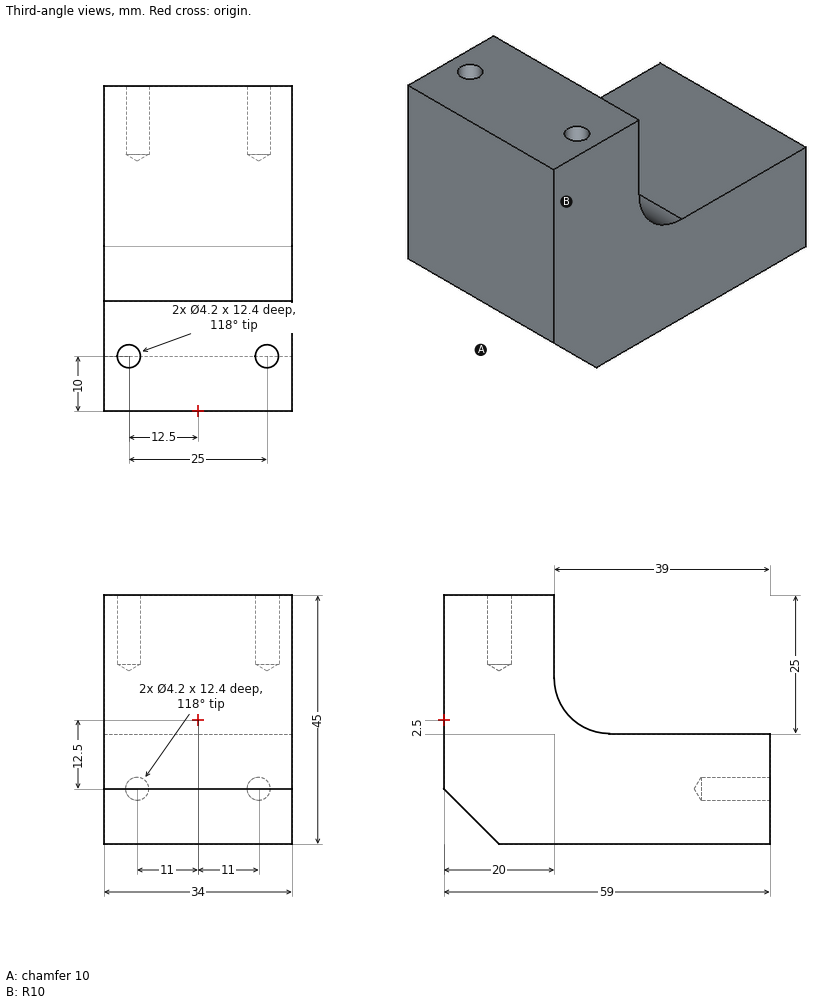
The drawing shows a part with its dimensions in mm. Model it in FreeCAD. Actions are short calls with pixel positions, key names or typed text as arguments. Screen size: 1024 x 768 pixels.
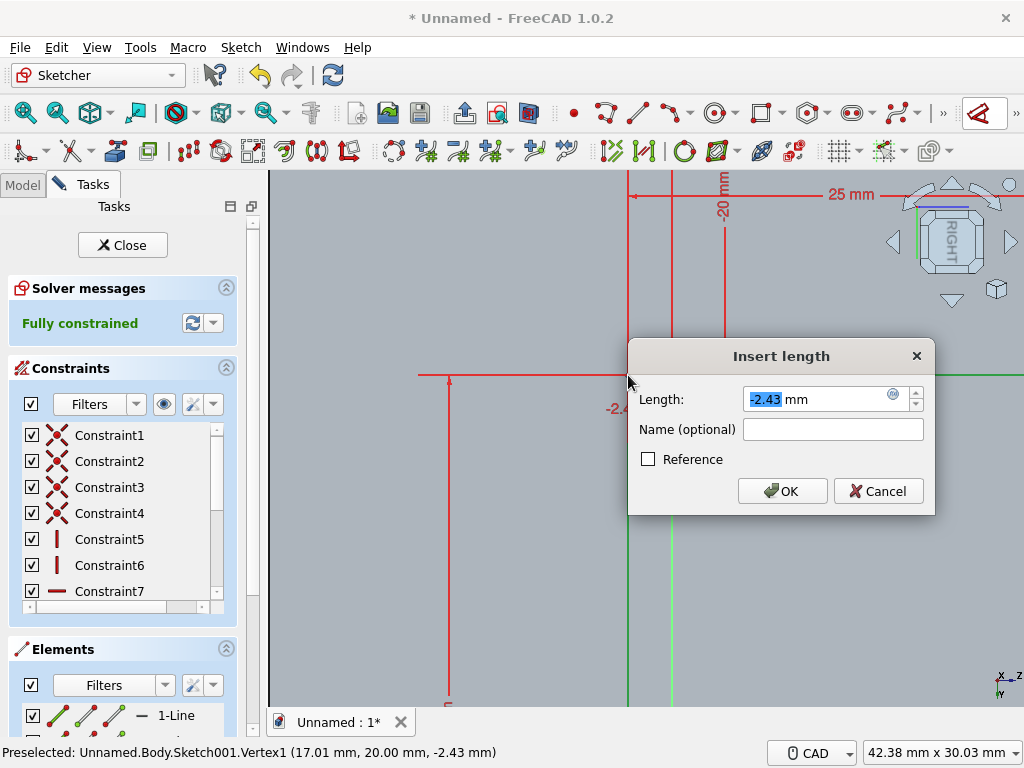
text(-2.5)
key(Return)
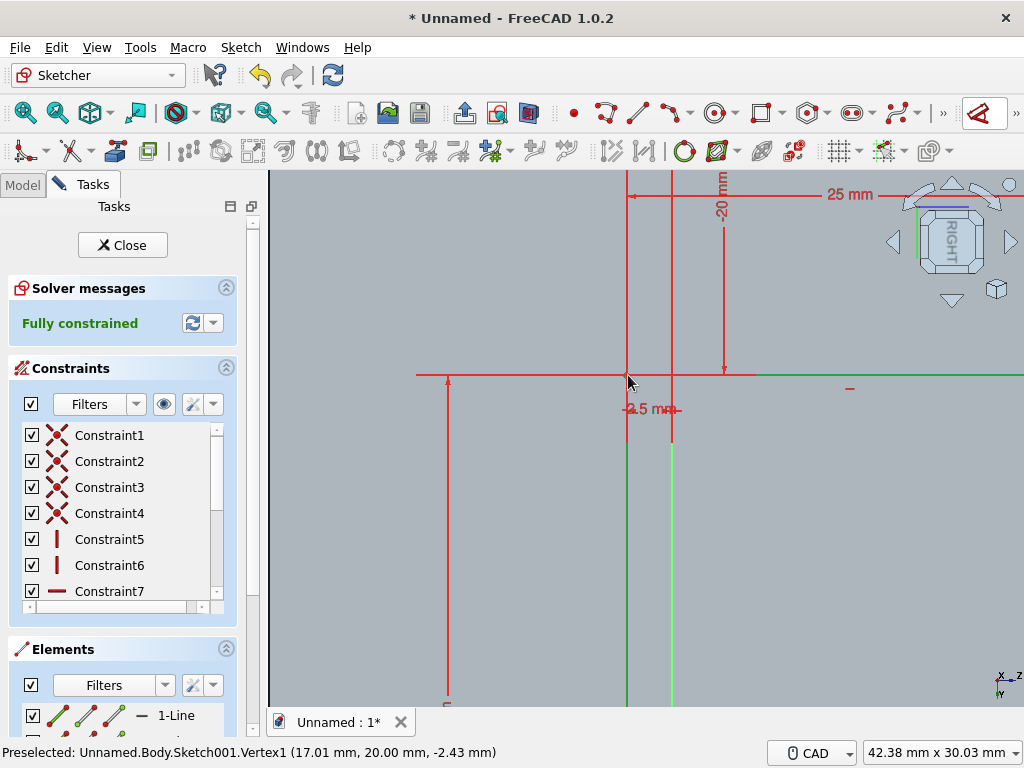
click(123, 245)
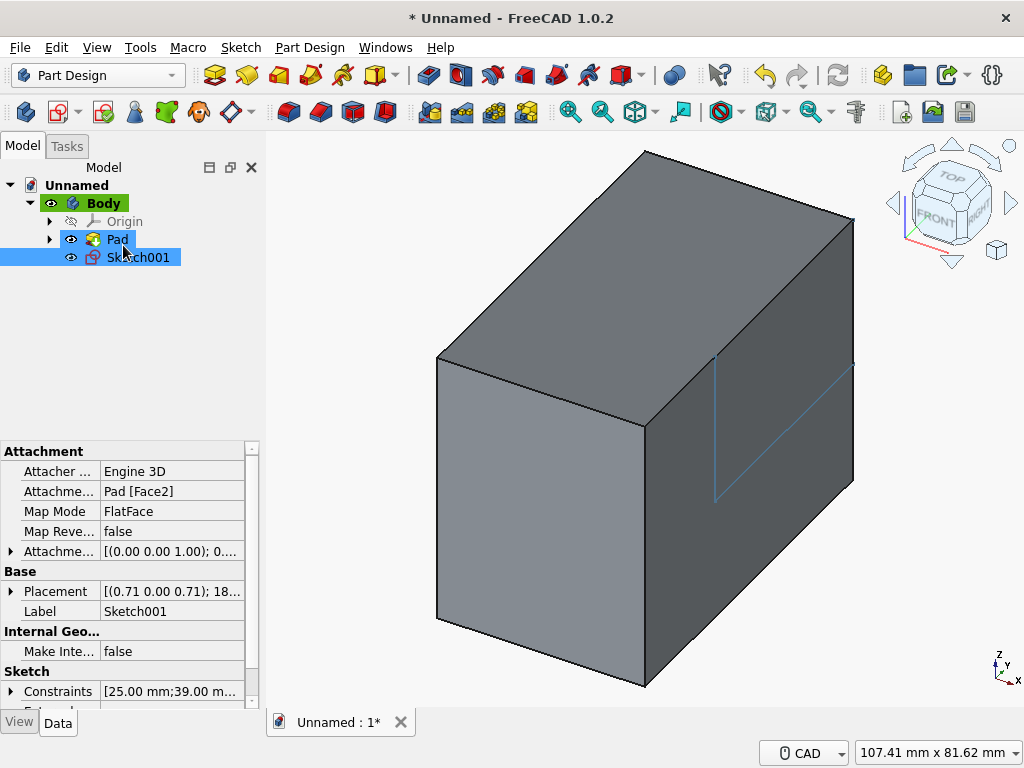
click(430, 76)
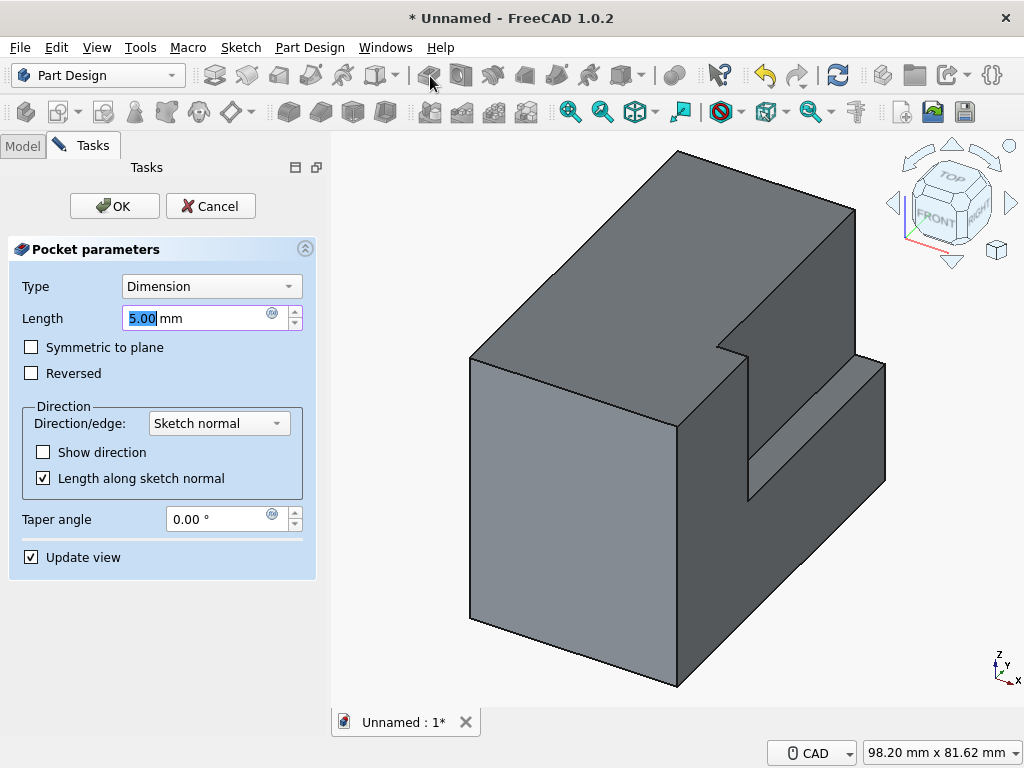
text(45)
key(Tab)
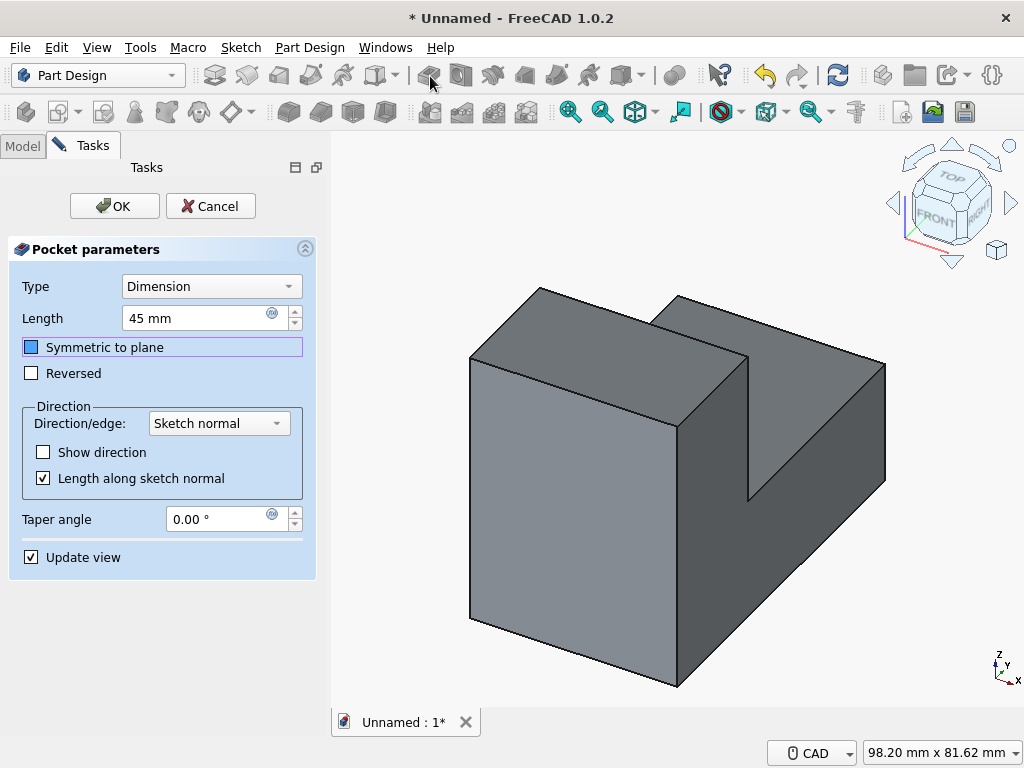
click(115, 206)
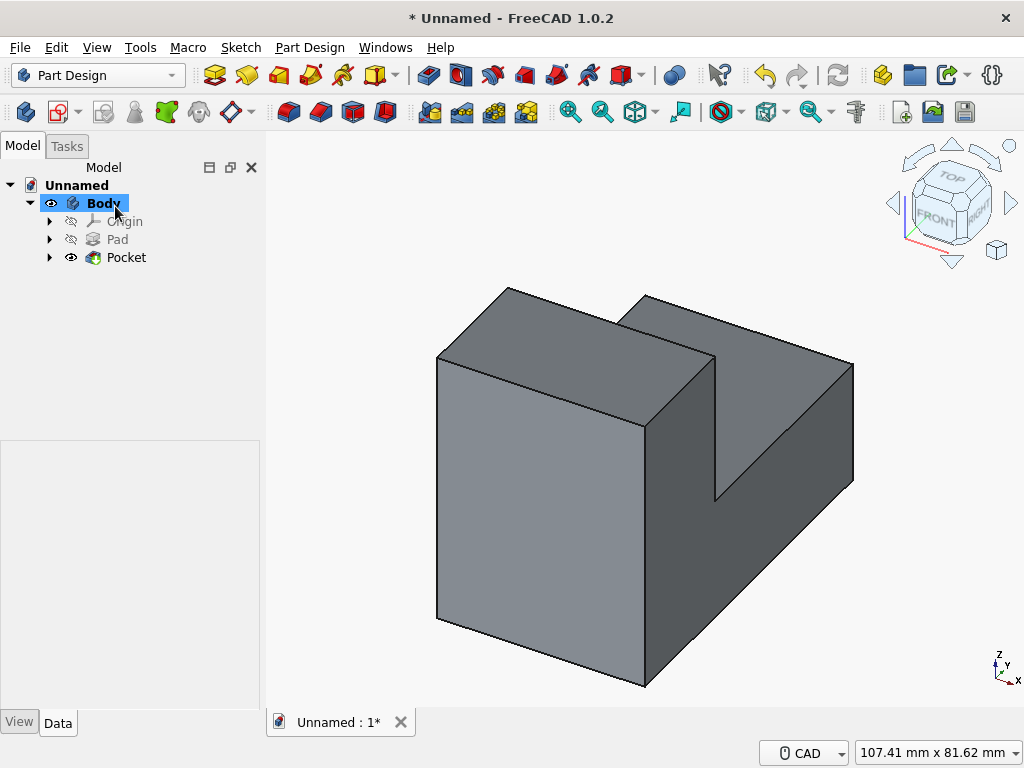
key(0)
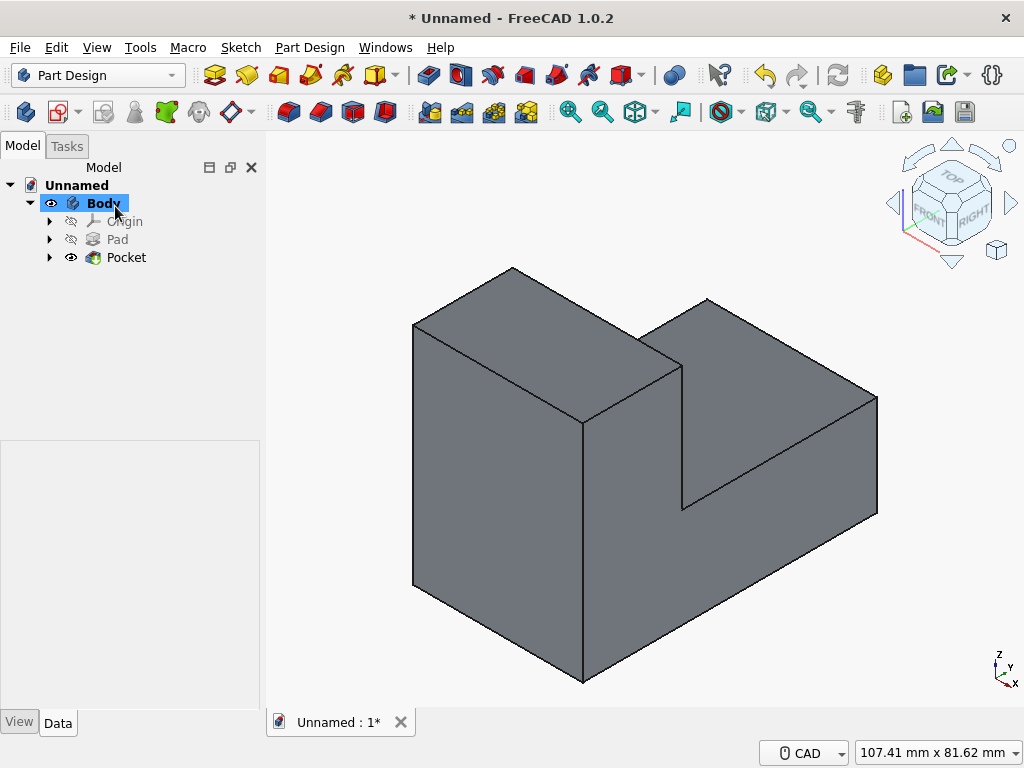
key(2)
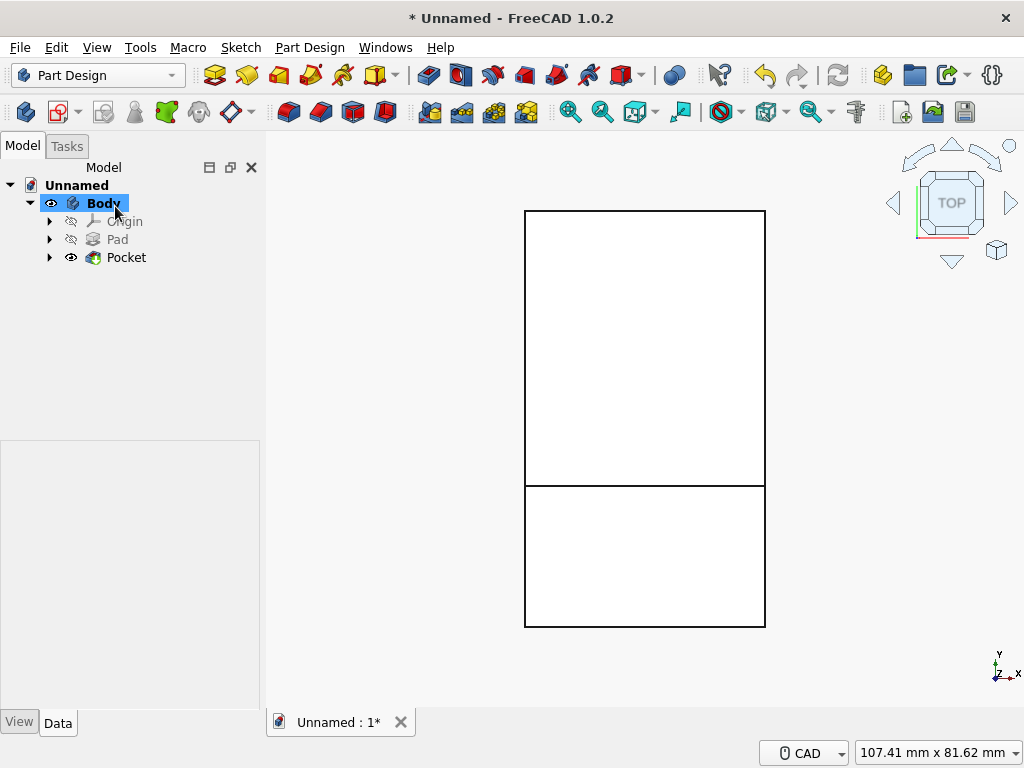
key(1)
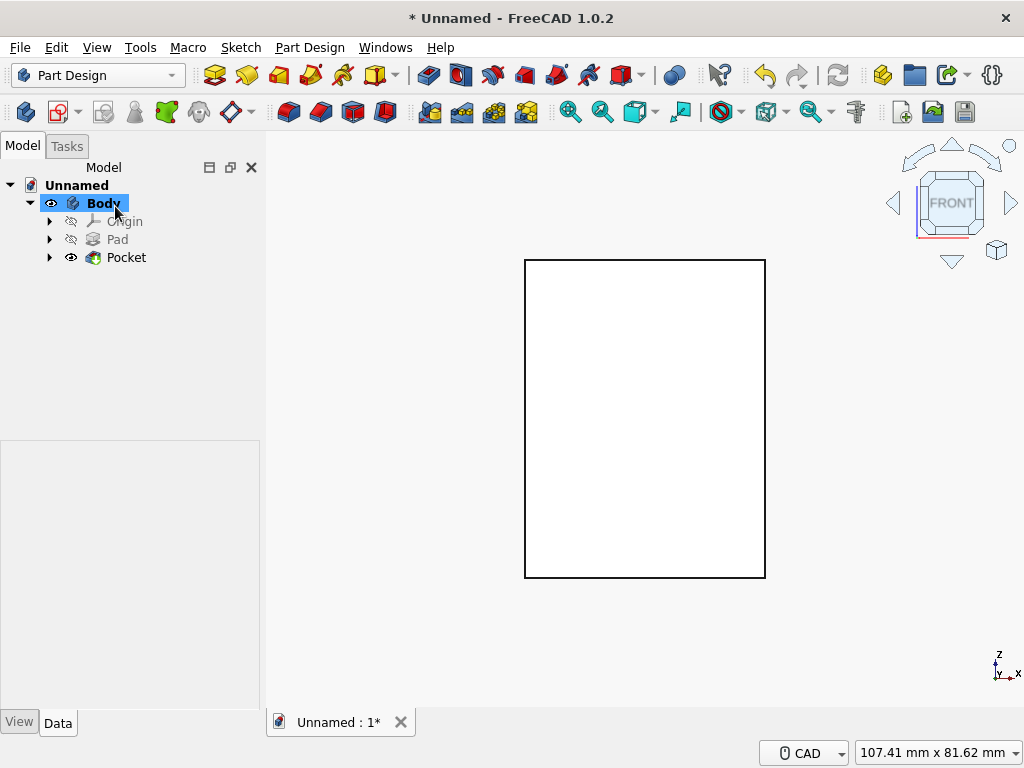
key(3)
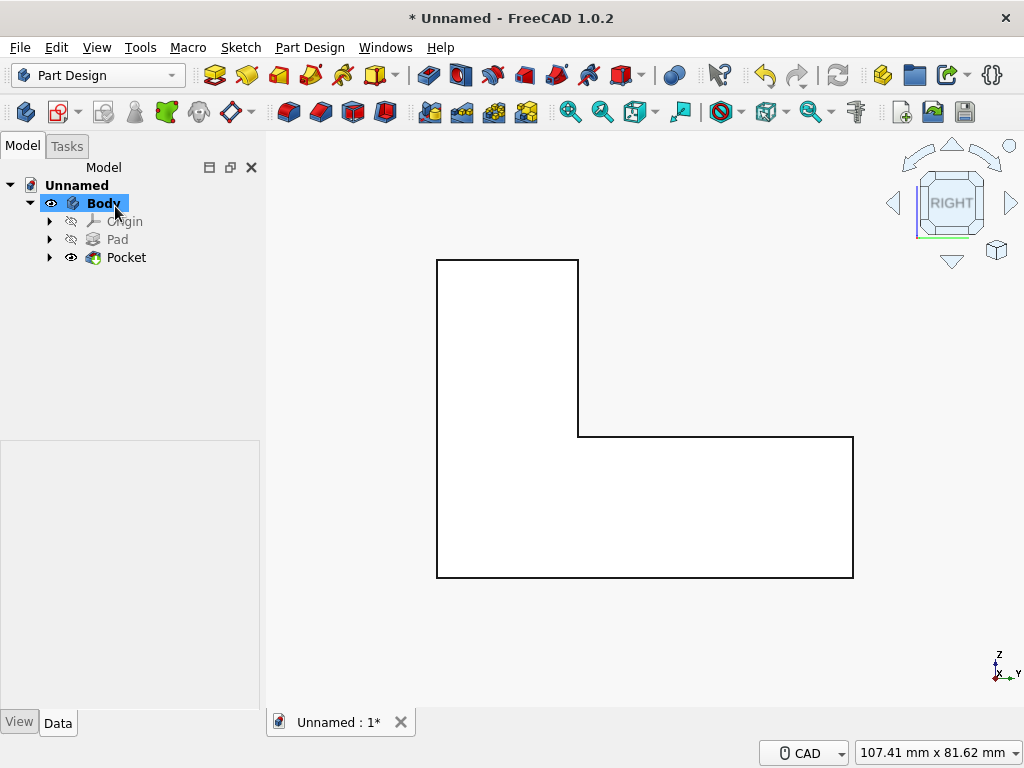
key(5)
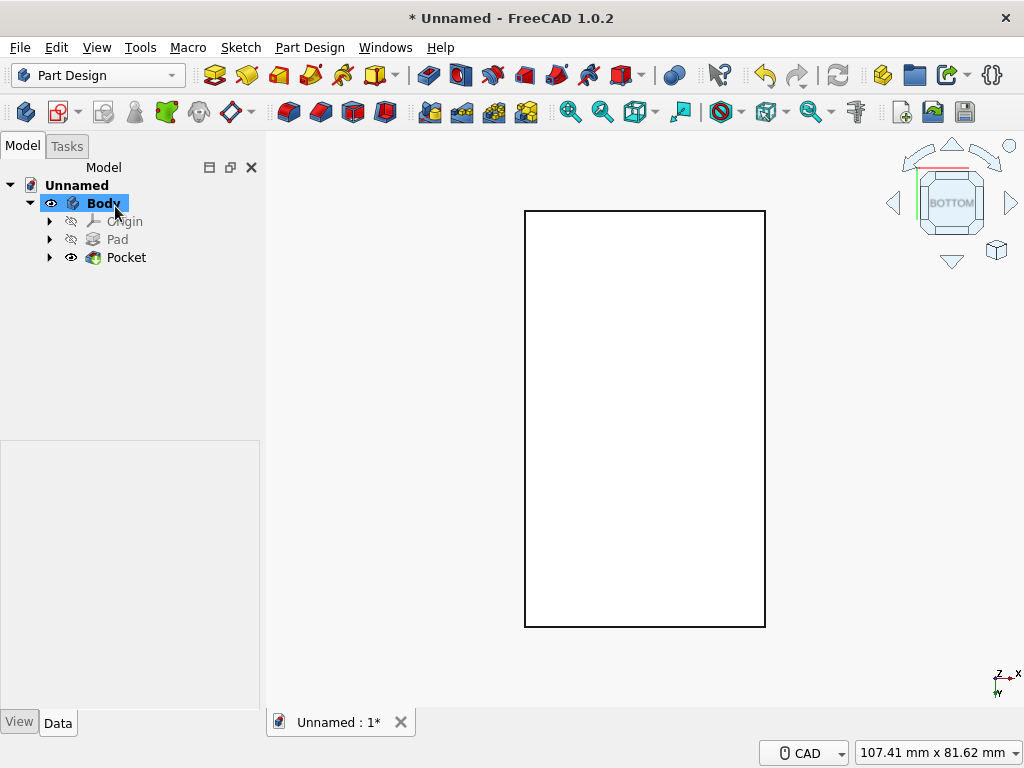
click(645, 210)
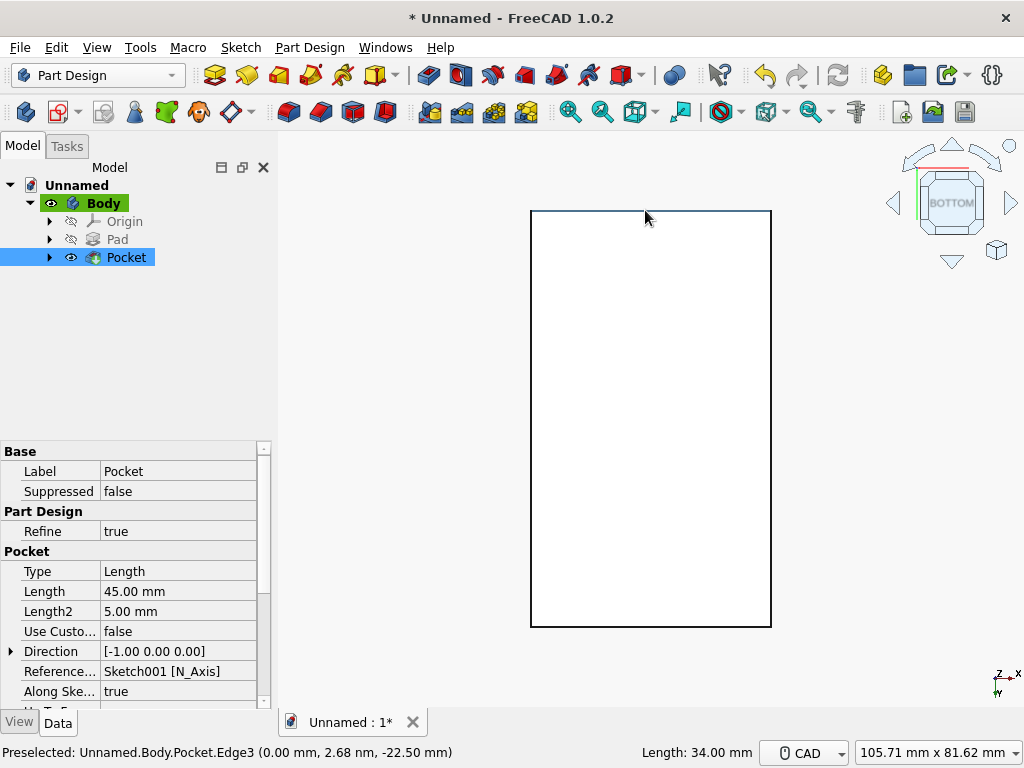
click(322, 112)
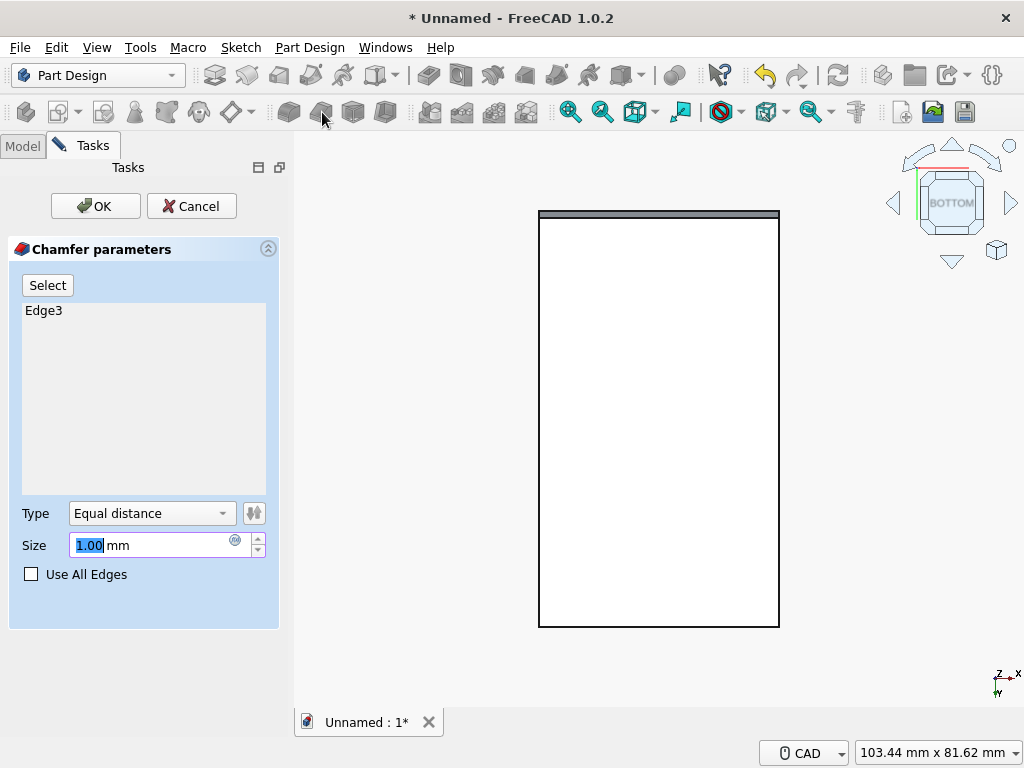
text(10)
key(Tab)